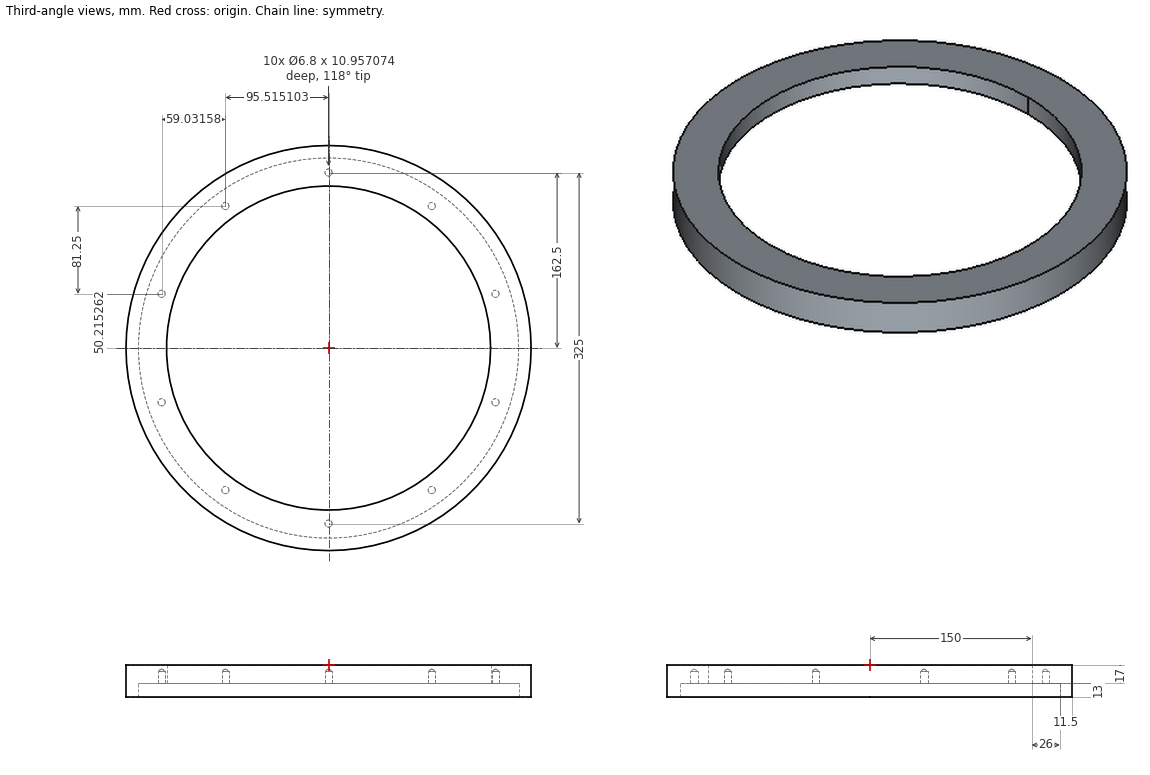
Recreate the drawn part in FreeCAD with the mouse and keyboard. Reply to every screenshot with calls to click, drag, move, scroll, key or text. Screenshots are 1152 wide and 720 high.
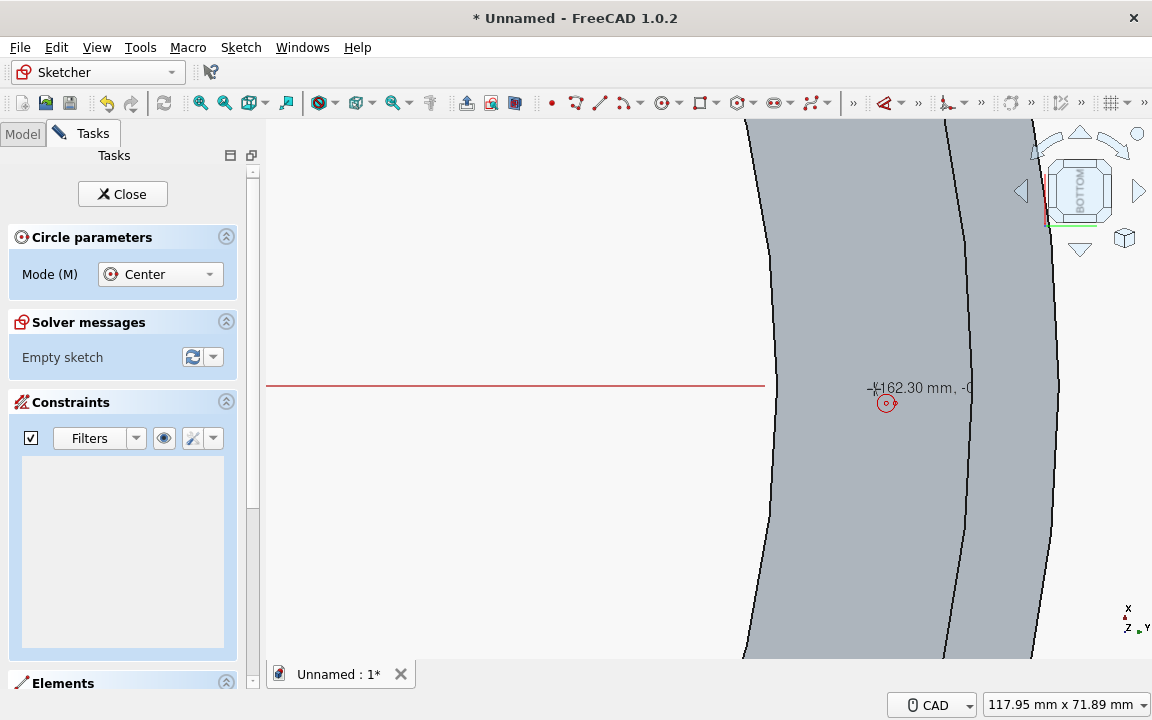
scroll(795, 390, down, 10)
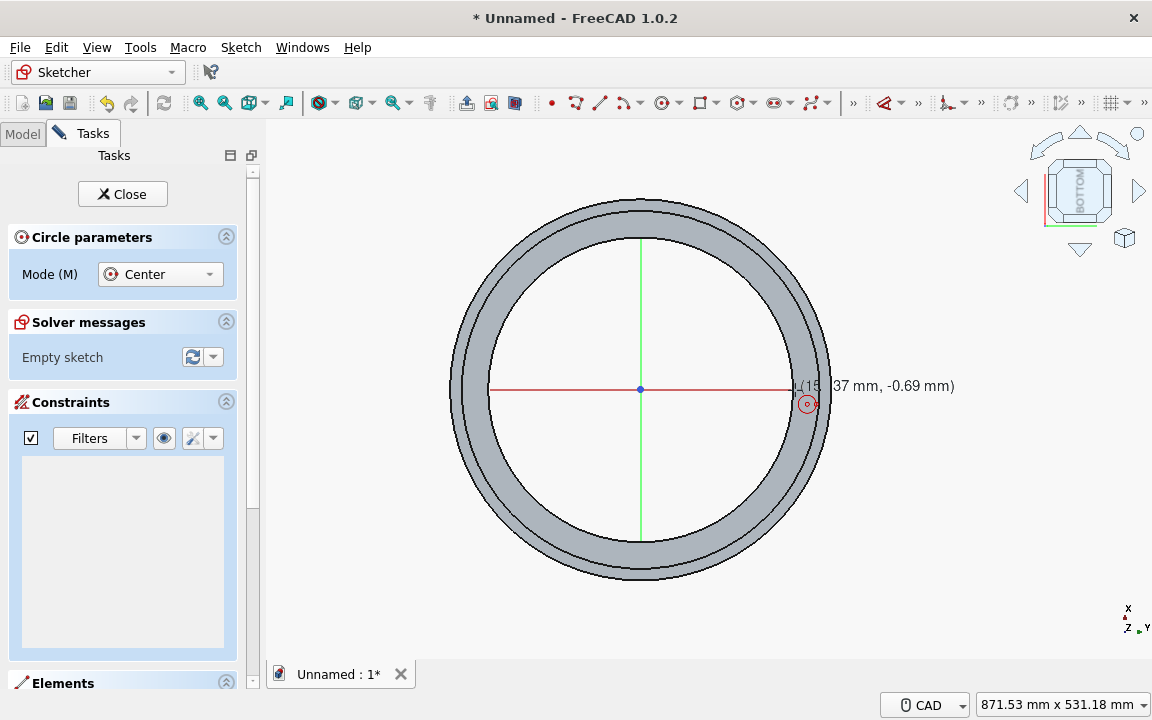
click(806, 390)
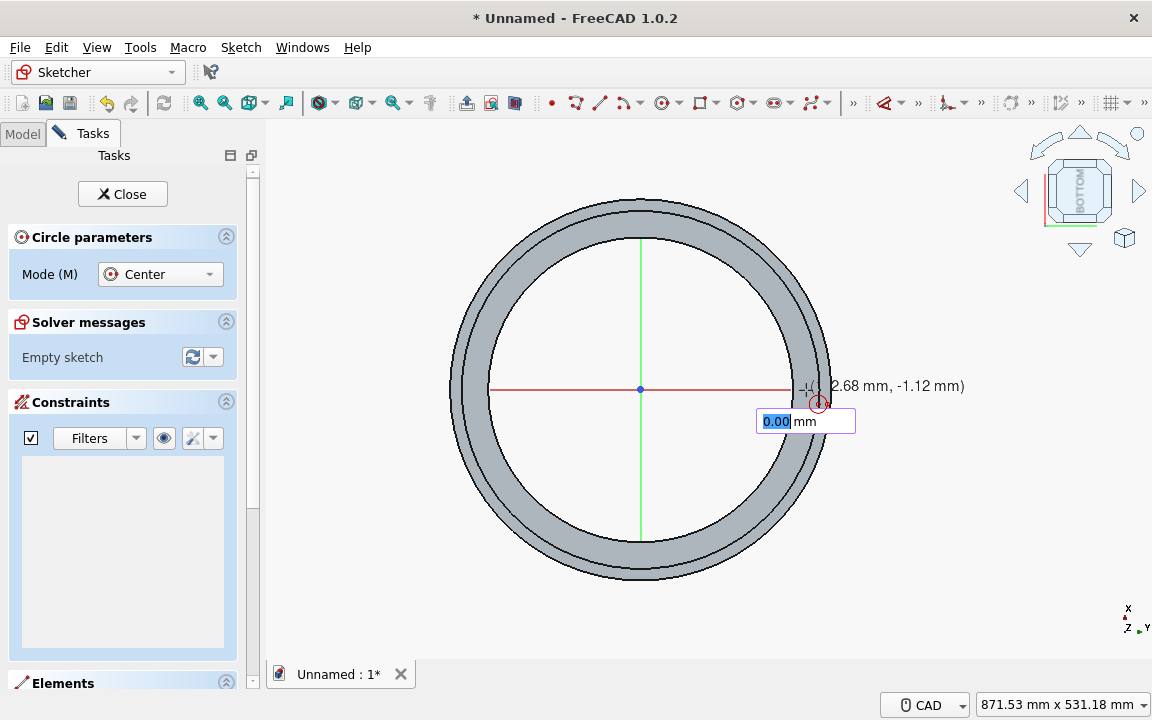
scroll(805, 393, up, 8)
move(801, 392)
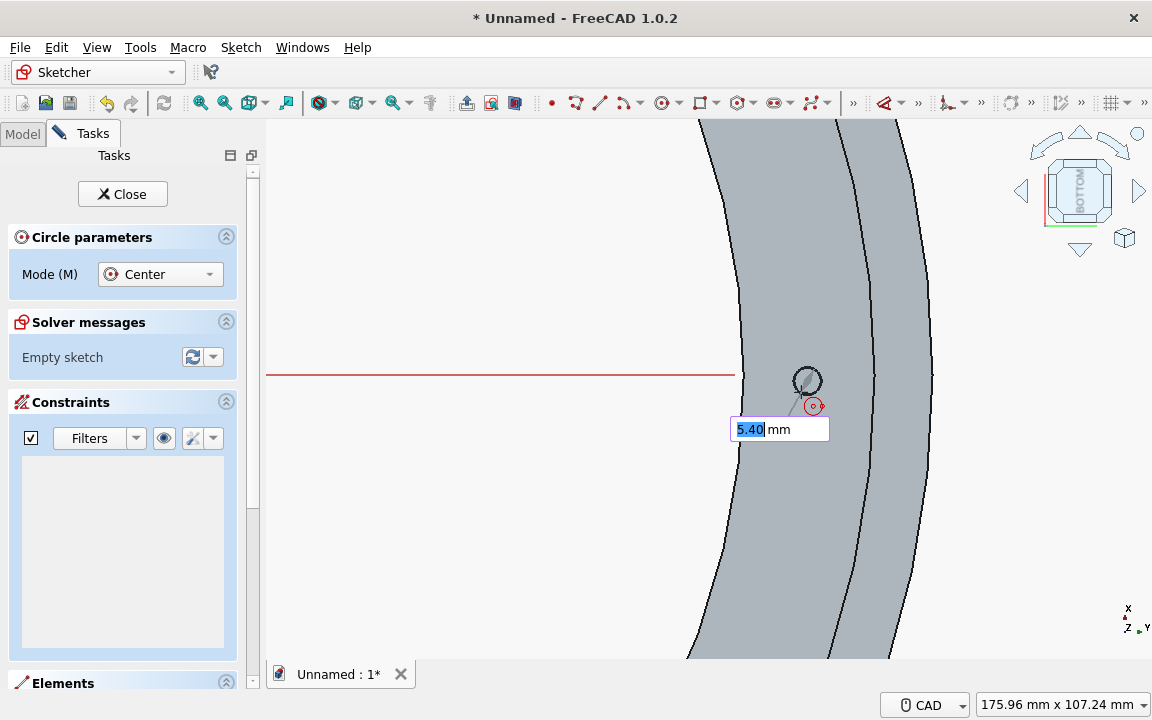
text(6.8)
key(Return)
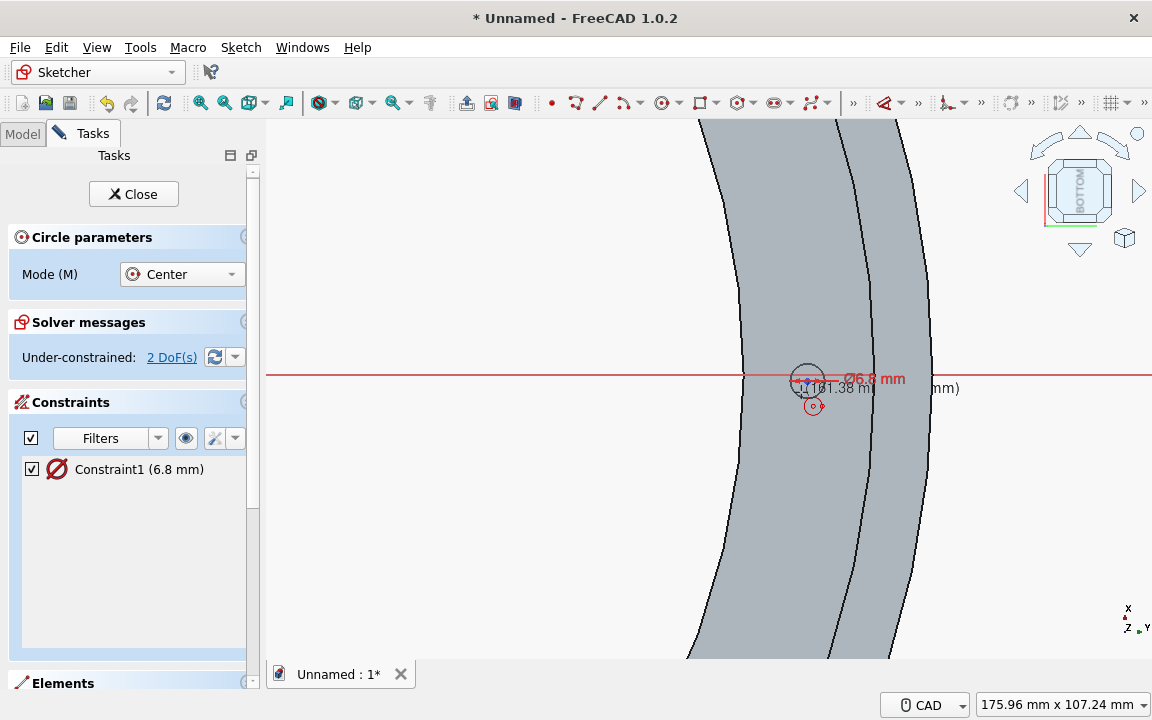
scroll(805, 392, down, 8)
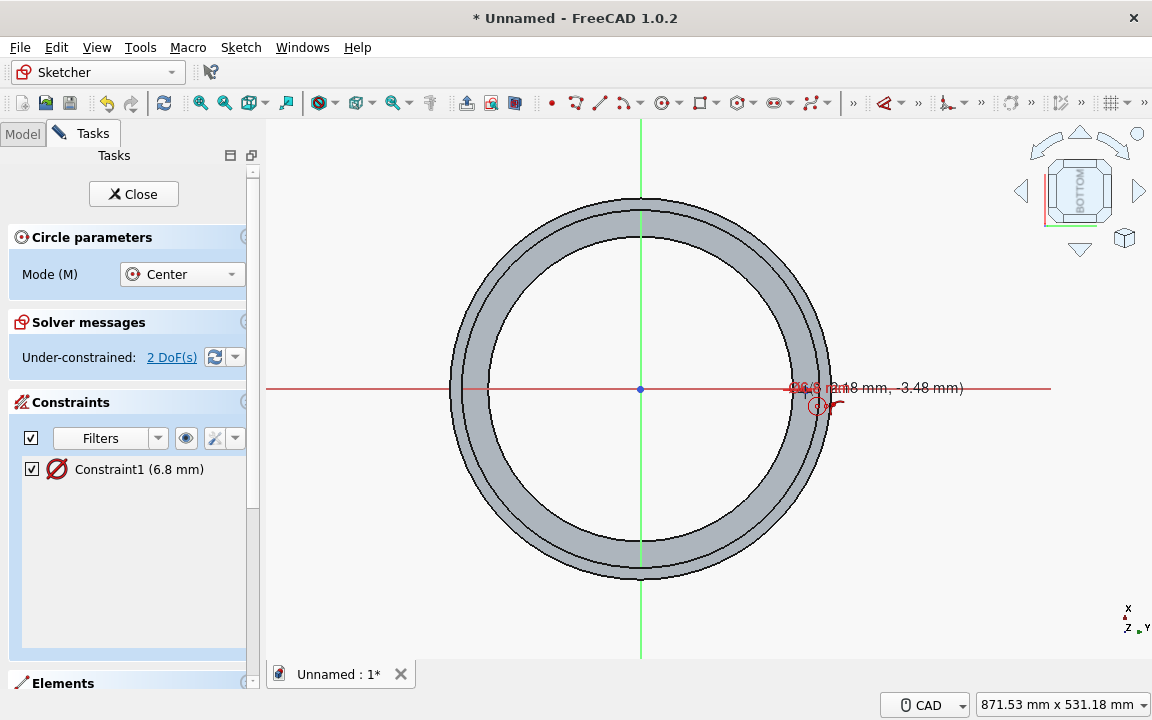
scroll(774, 486, up, 10)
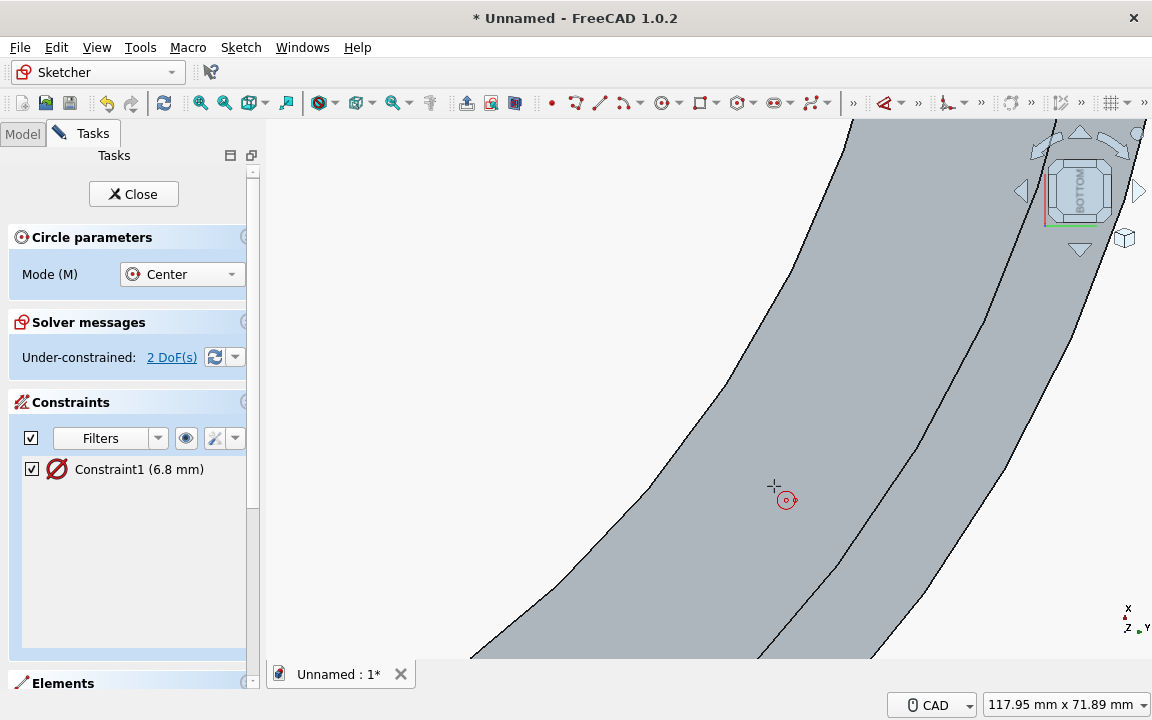
scroll(774, 487, down, 10)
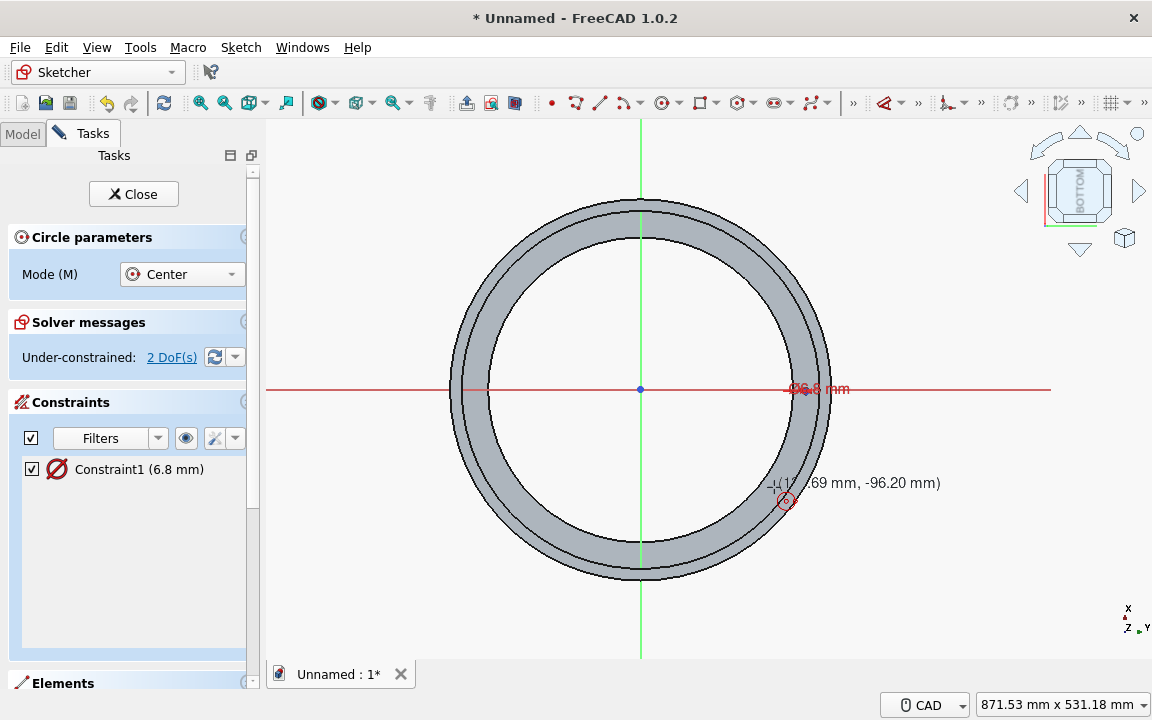
click(774, 487)
move(777, 485)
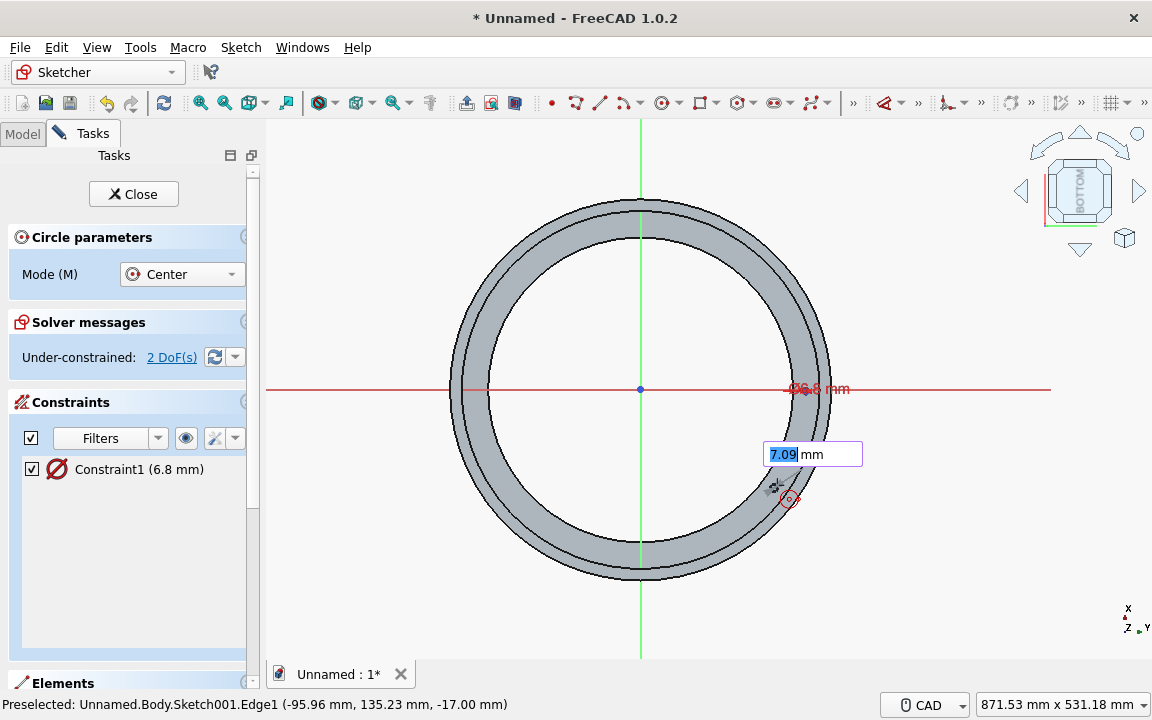
text(6.8)
key(Return)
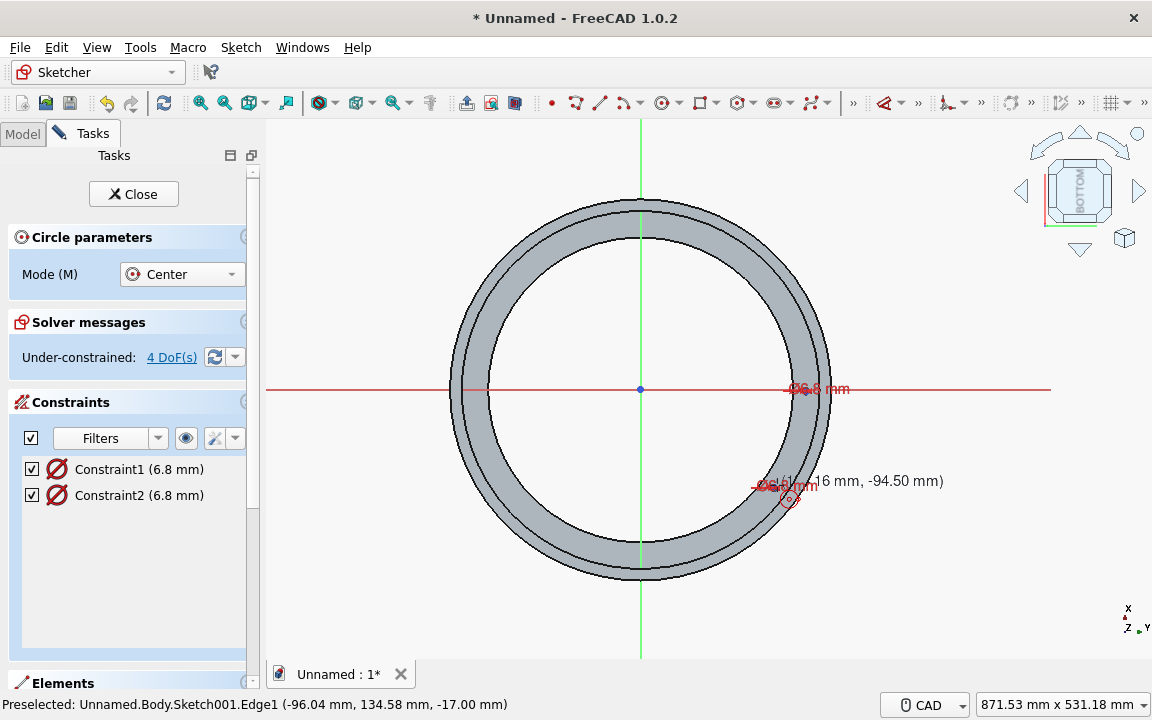
scroll(692, 547, up, 10)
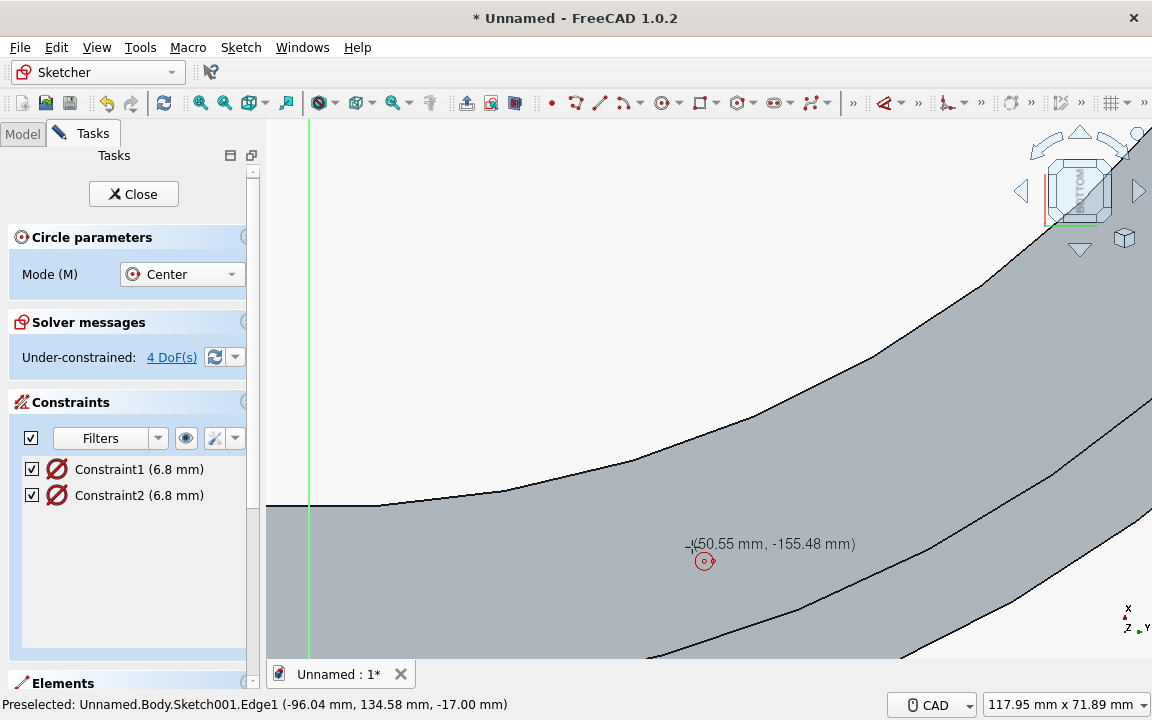
scroll(692, 547, down, 10)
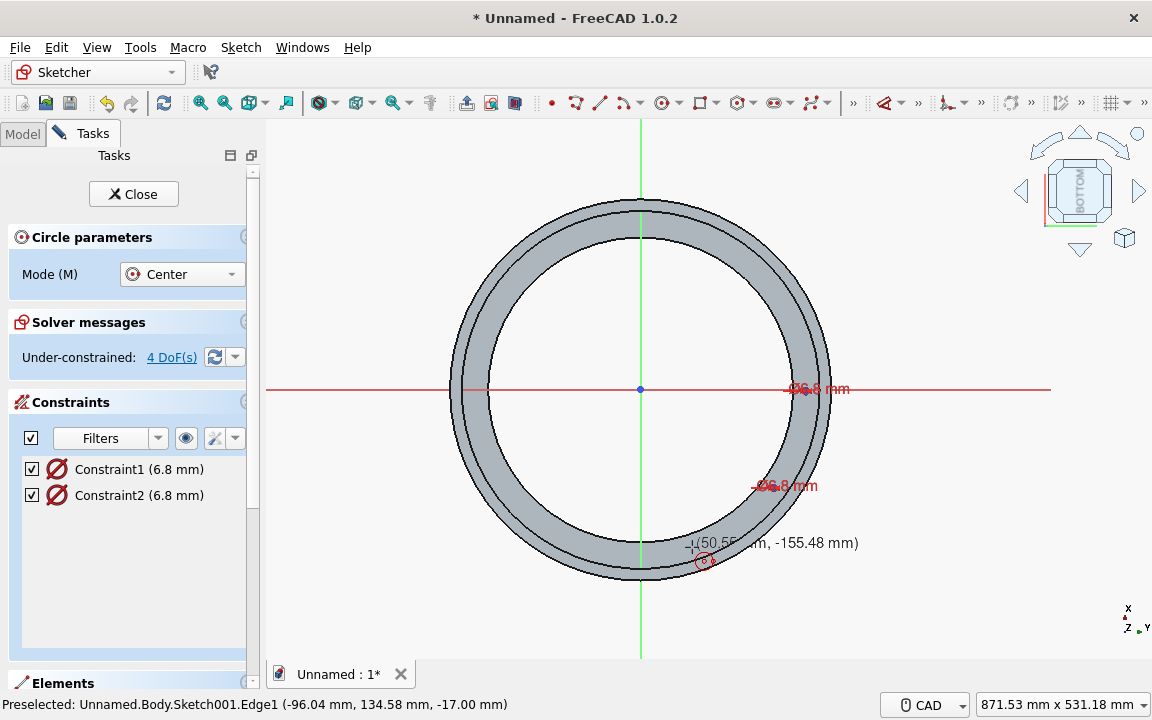
click(692, 547)
move(694, 545)